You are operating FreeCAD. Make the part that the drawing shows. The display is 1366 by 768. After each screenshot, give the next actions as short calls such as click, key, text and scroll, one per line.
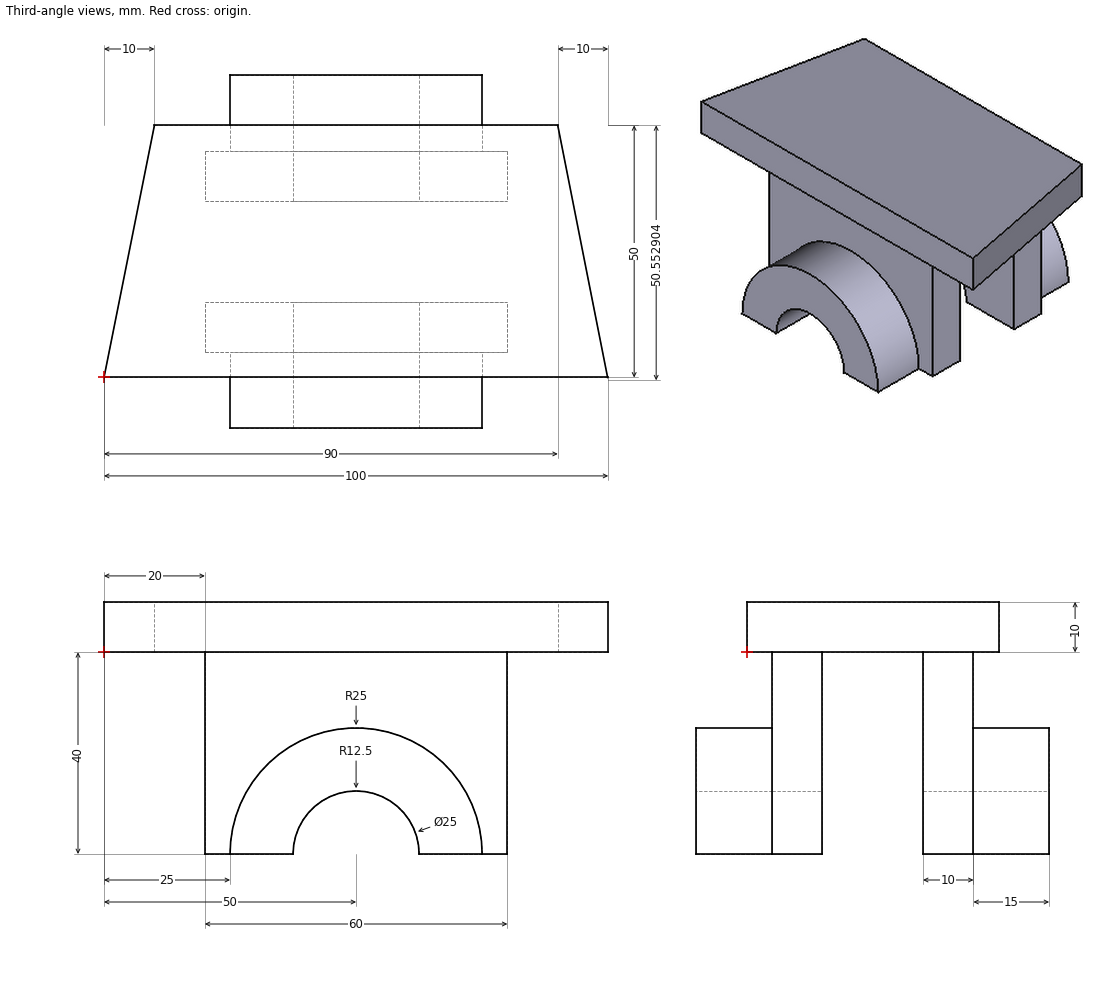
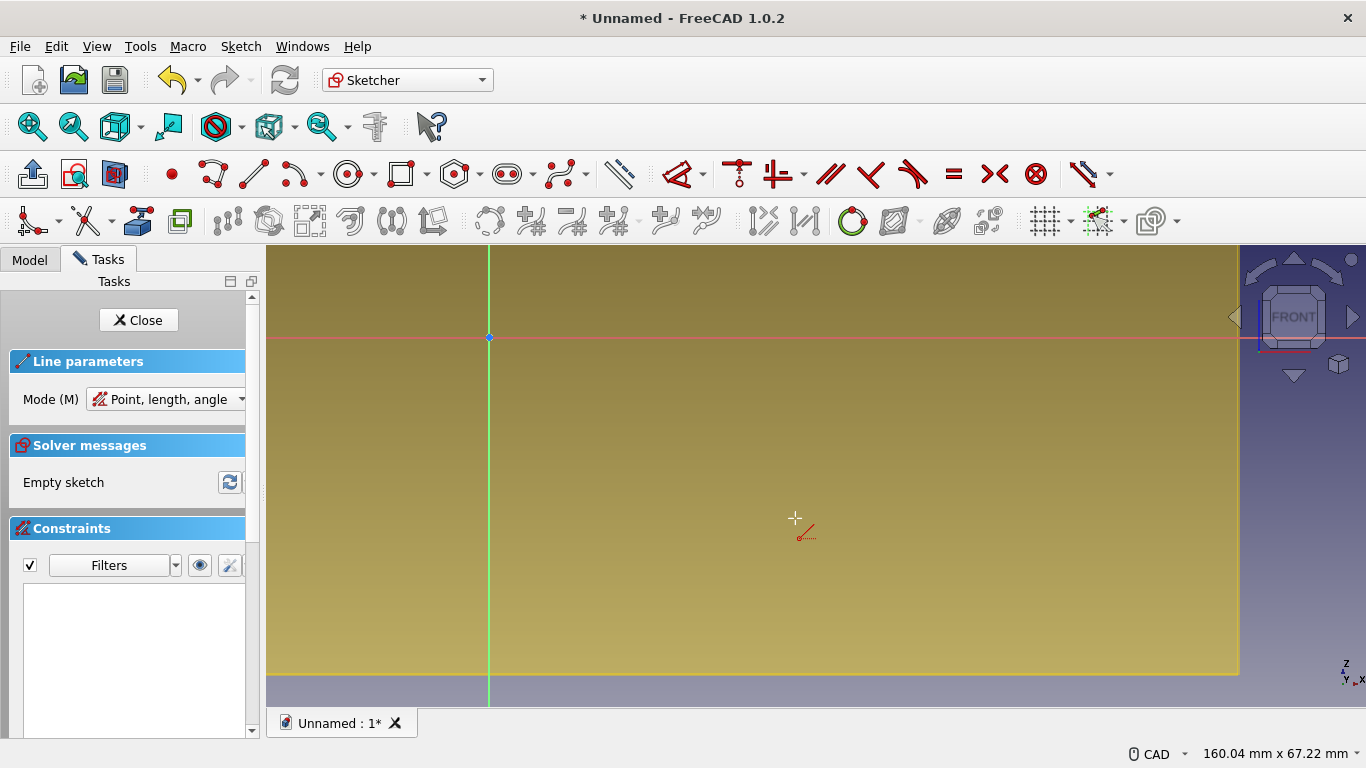
click(747, 613)
click(661, 613)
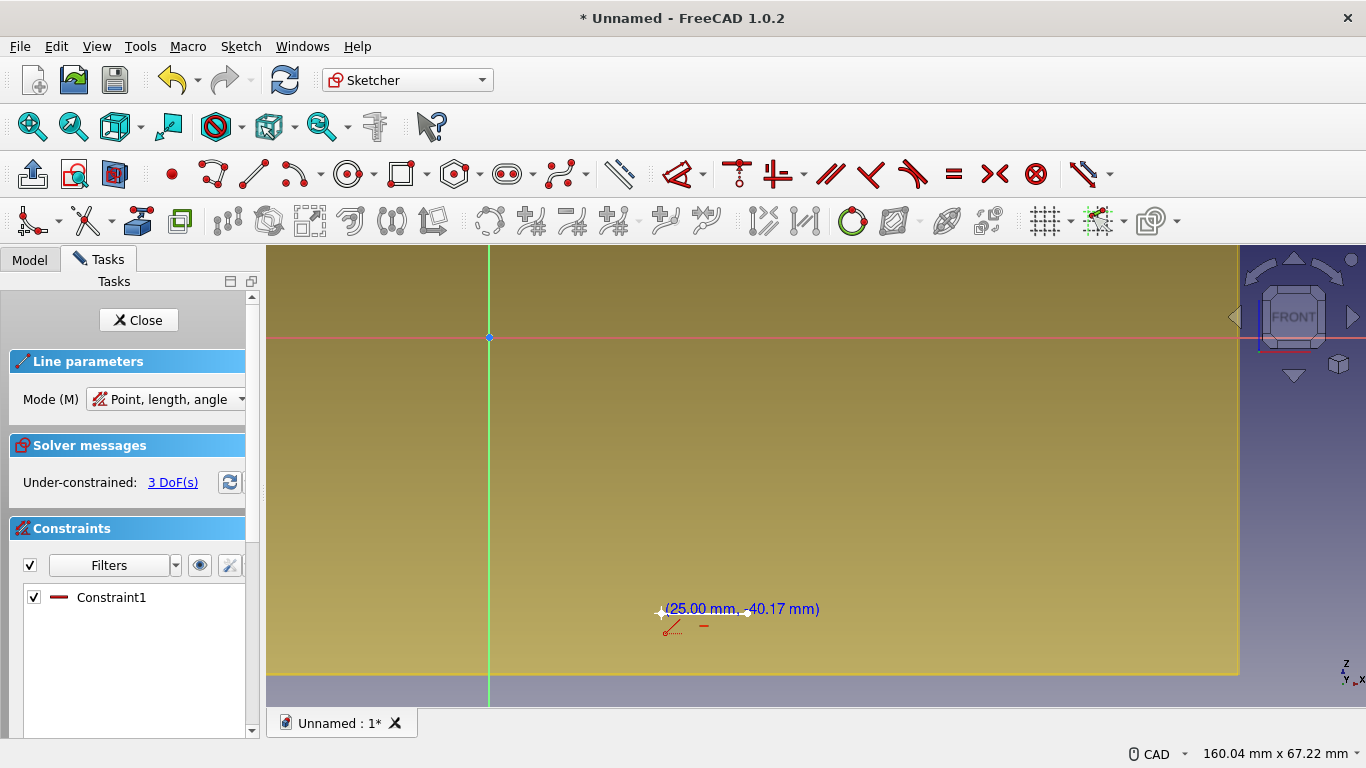
click(1005, 613)
click(919, 613)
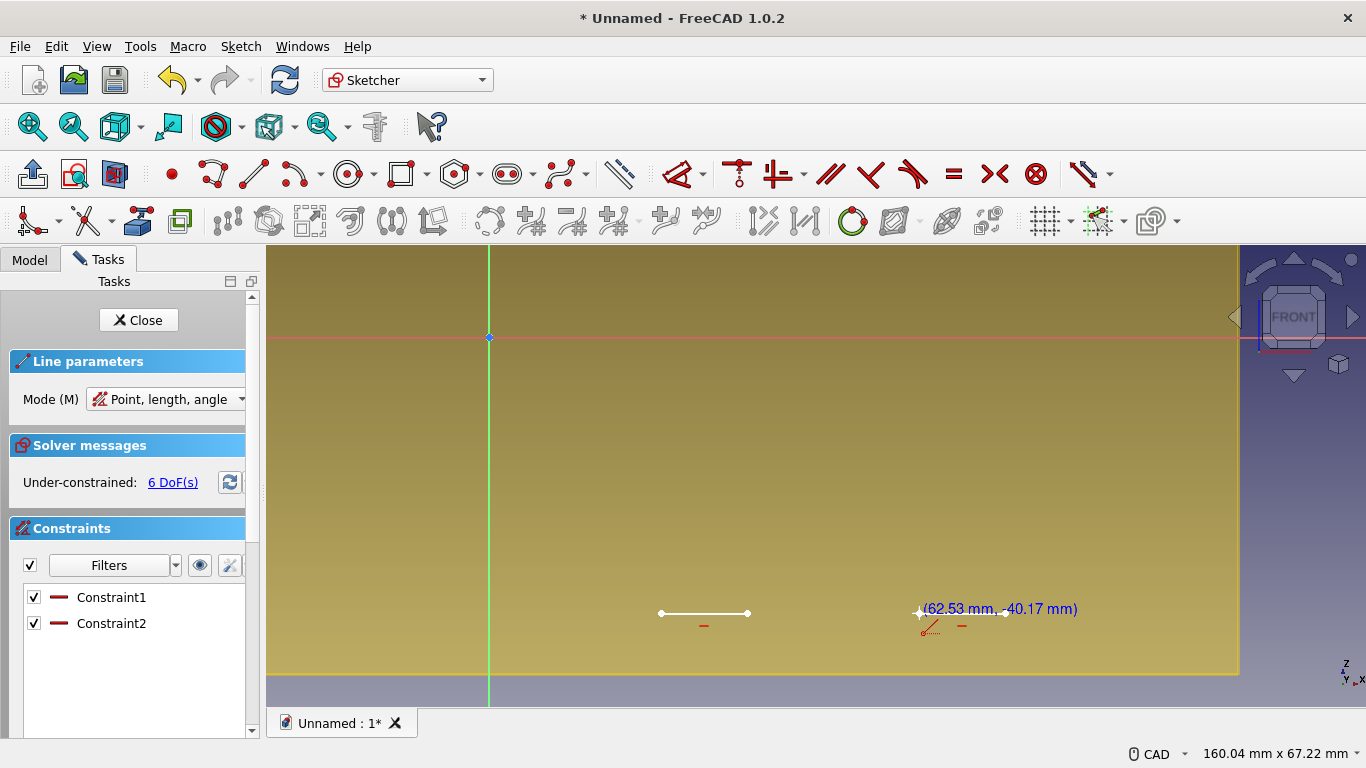
key(g)
key(3)
key(a)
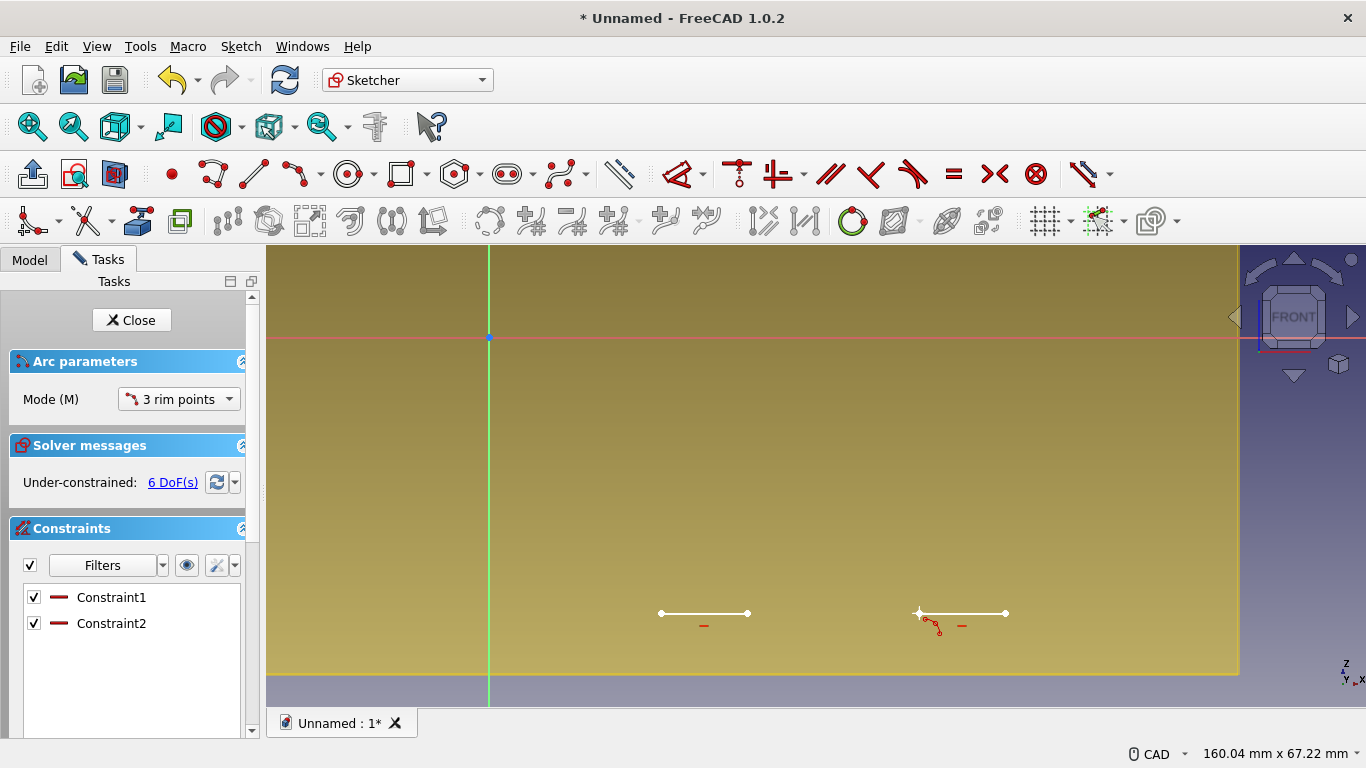
click(661, 614)
click(1005, 614)
click(833, 441)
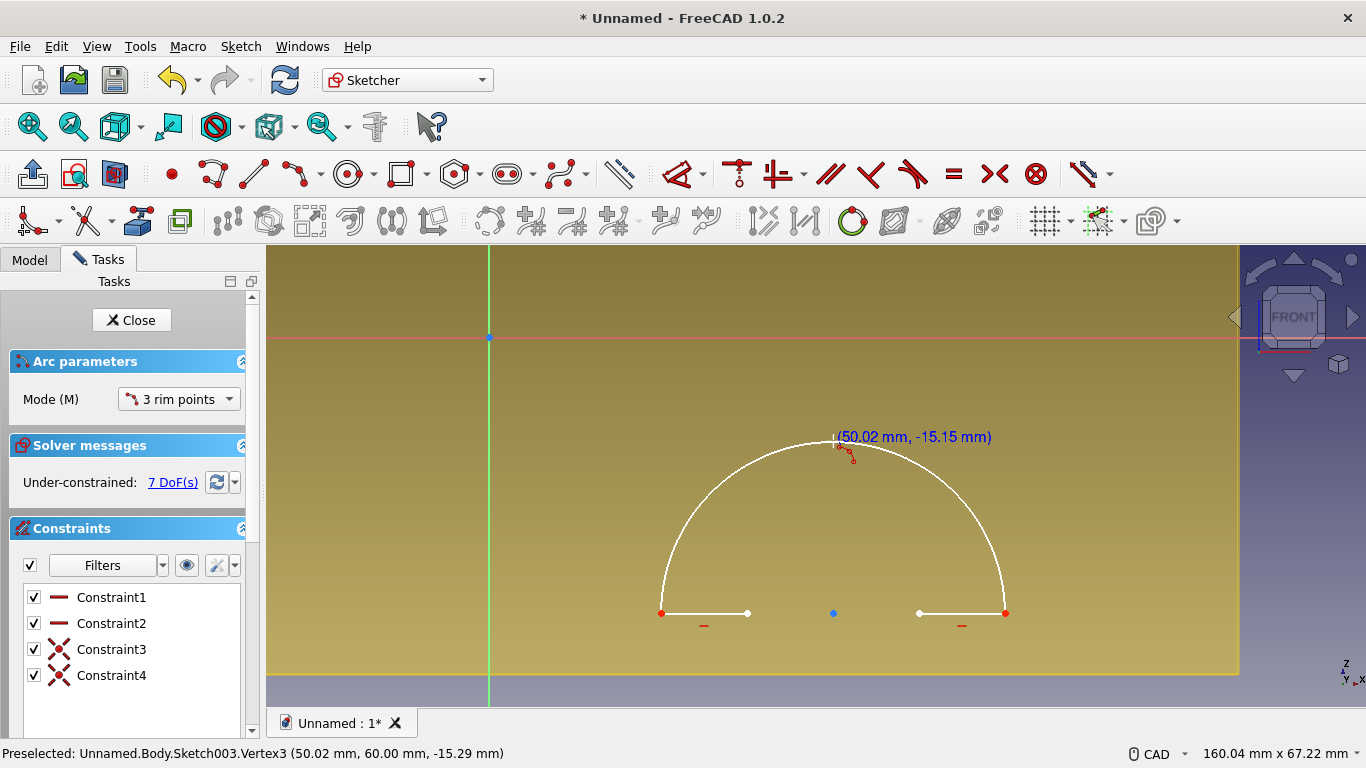
click(919, 614)
click(747, 614)
click(833, 527)
key(Escape)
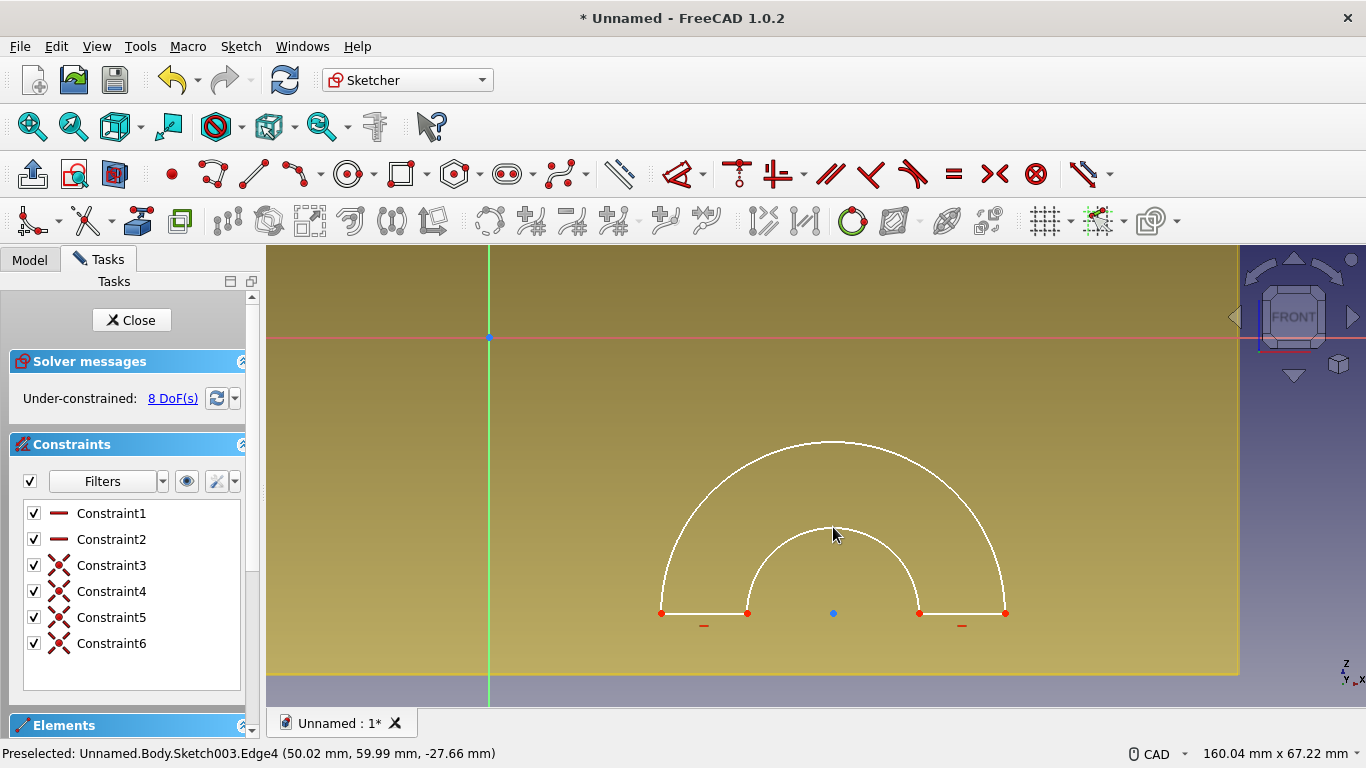
click(934, 475)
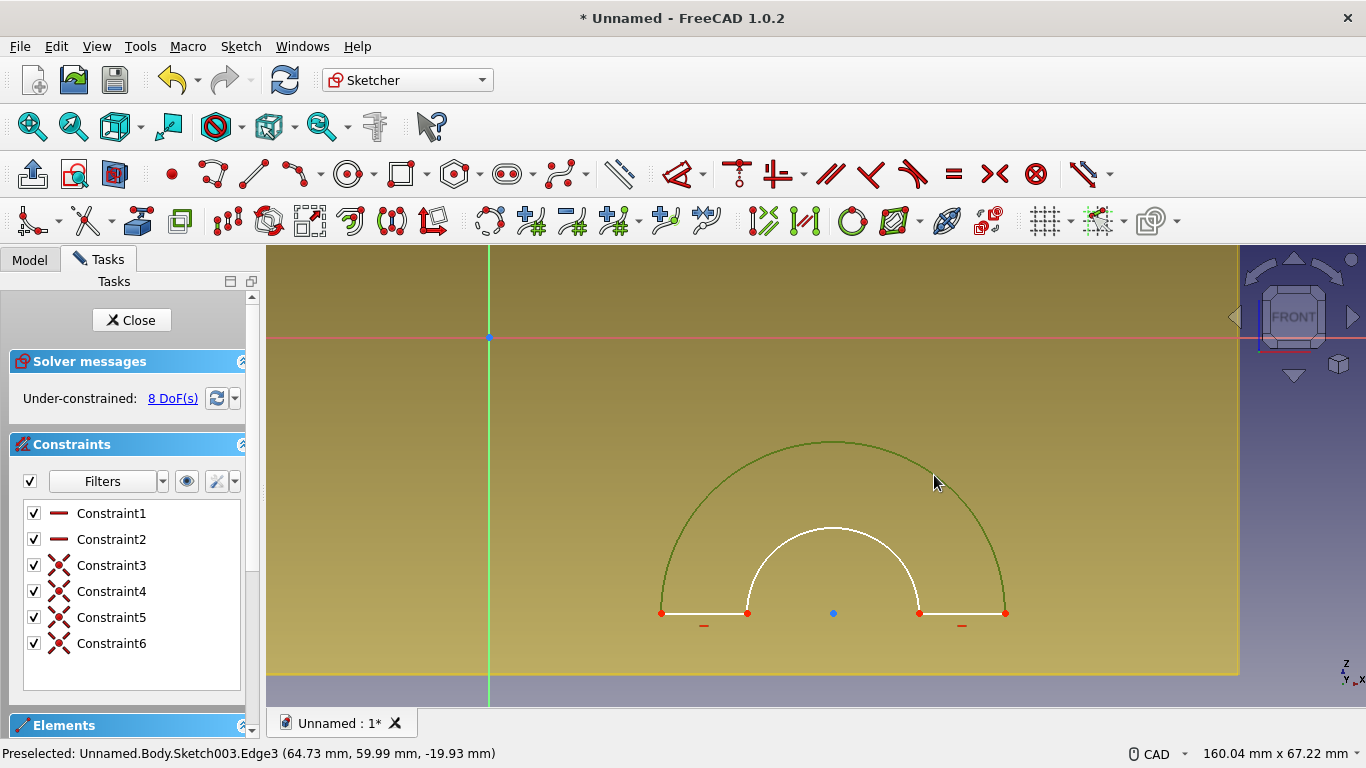
click(884, 544)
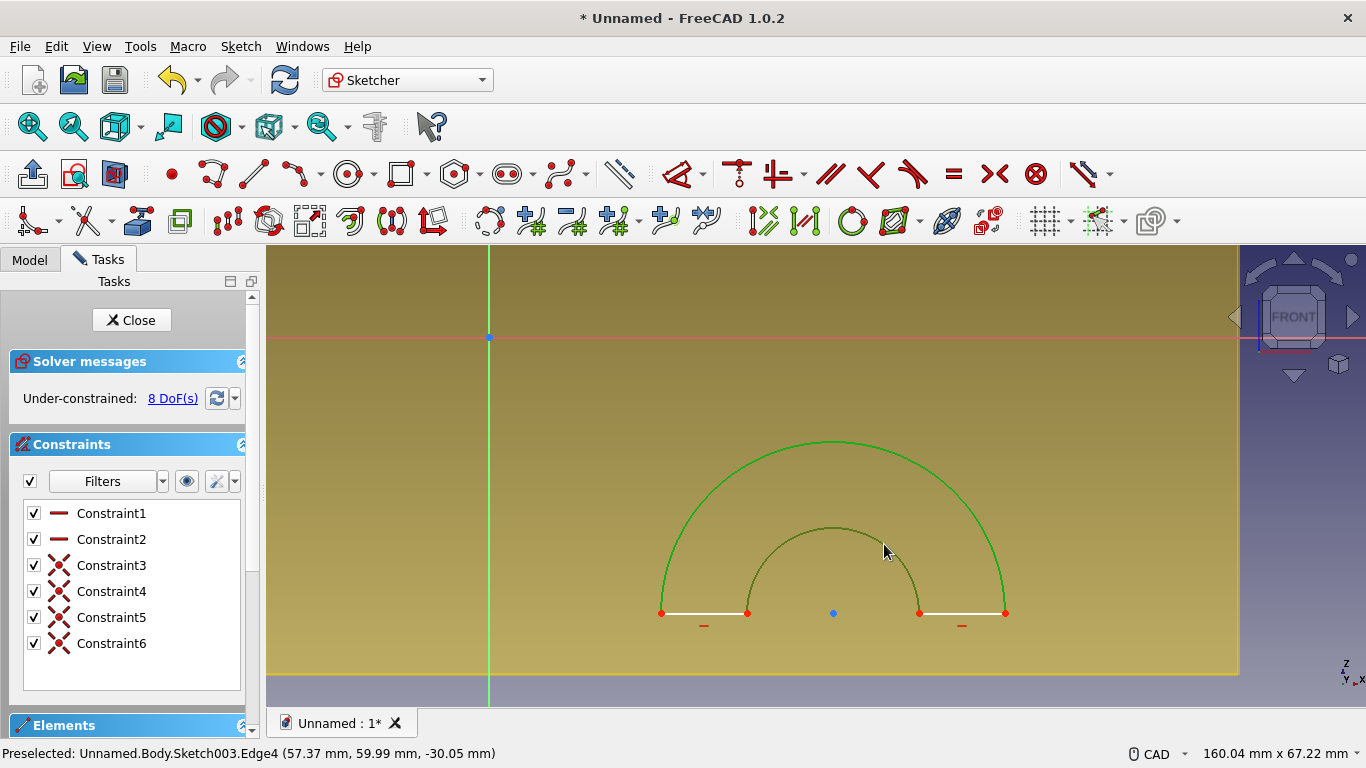
click(737, 174)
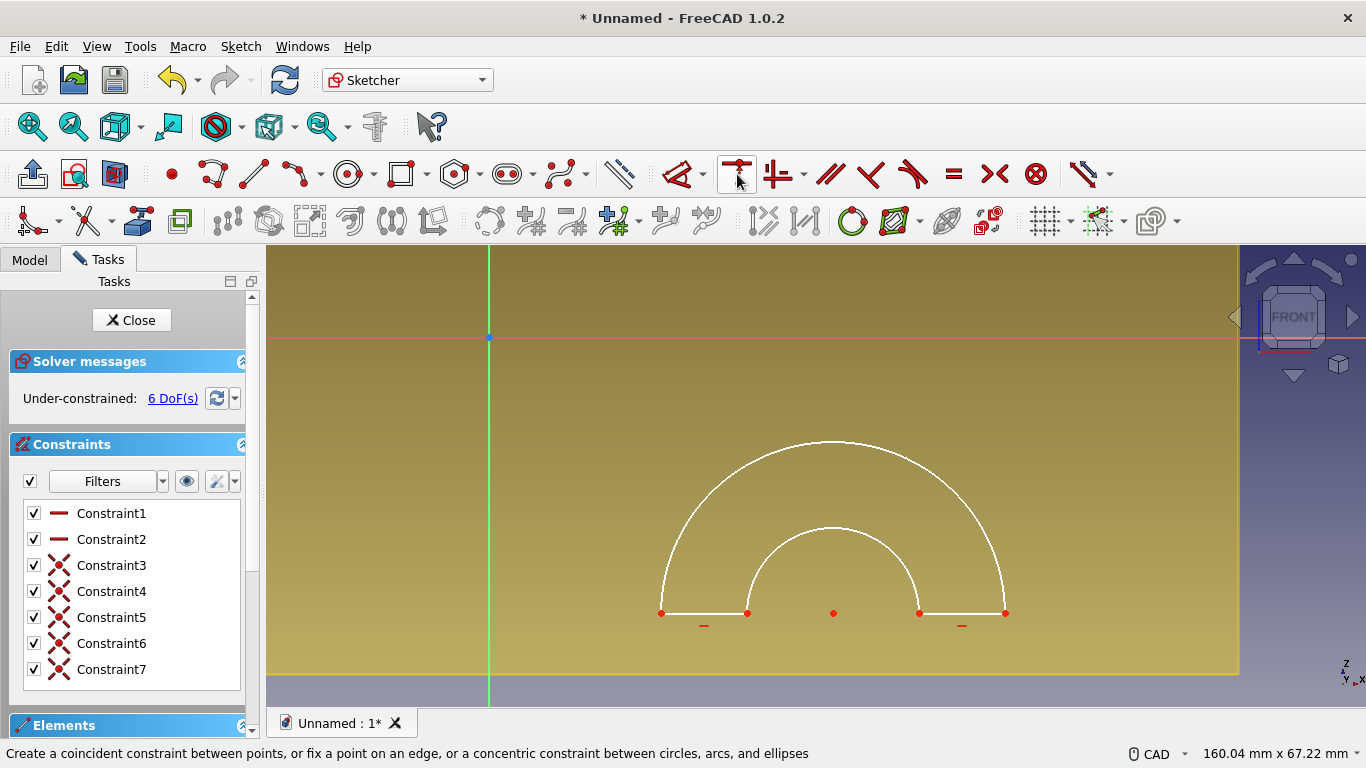
key(d)